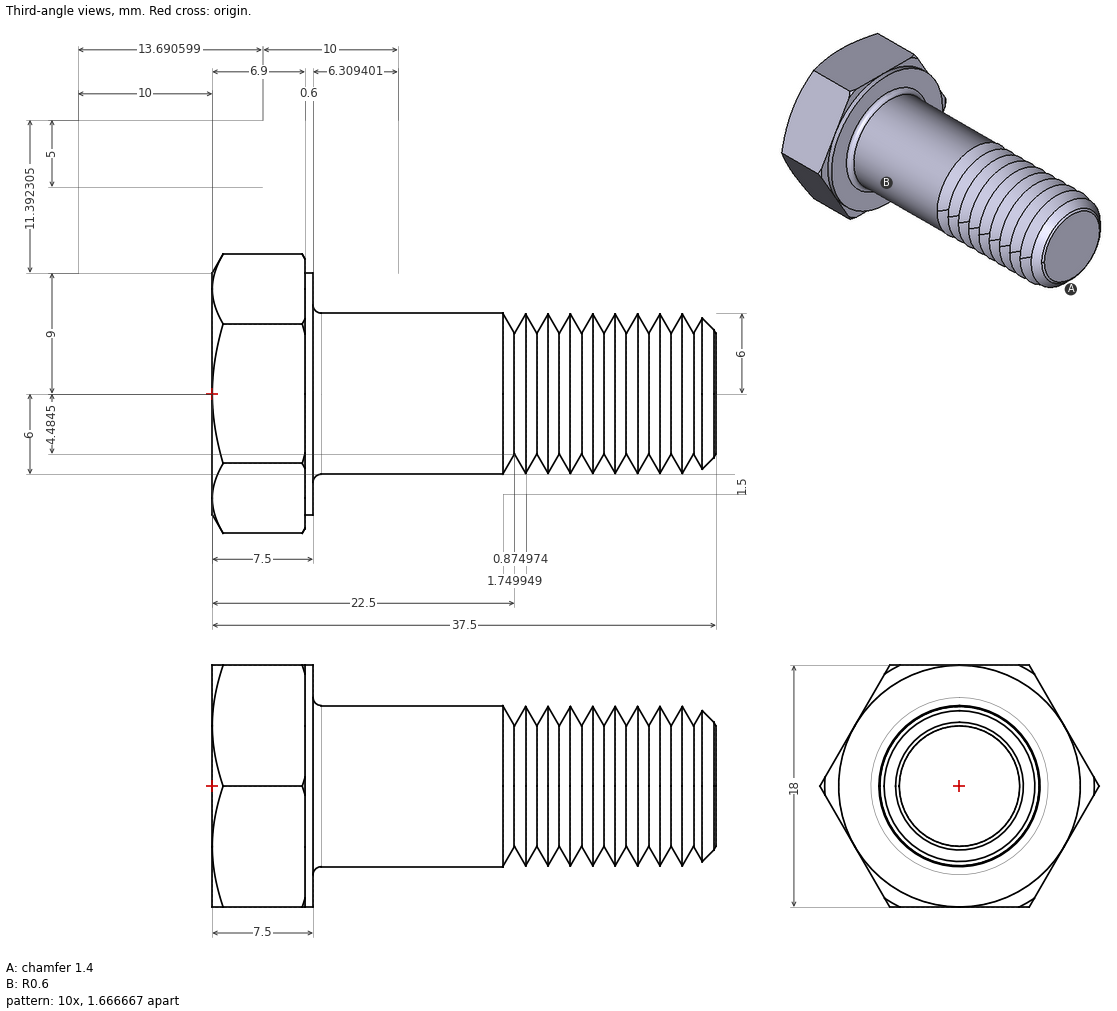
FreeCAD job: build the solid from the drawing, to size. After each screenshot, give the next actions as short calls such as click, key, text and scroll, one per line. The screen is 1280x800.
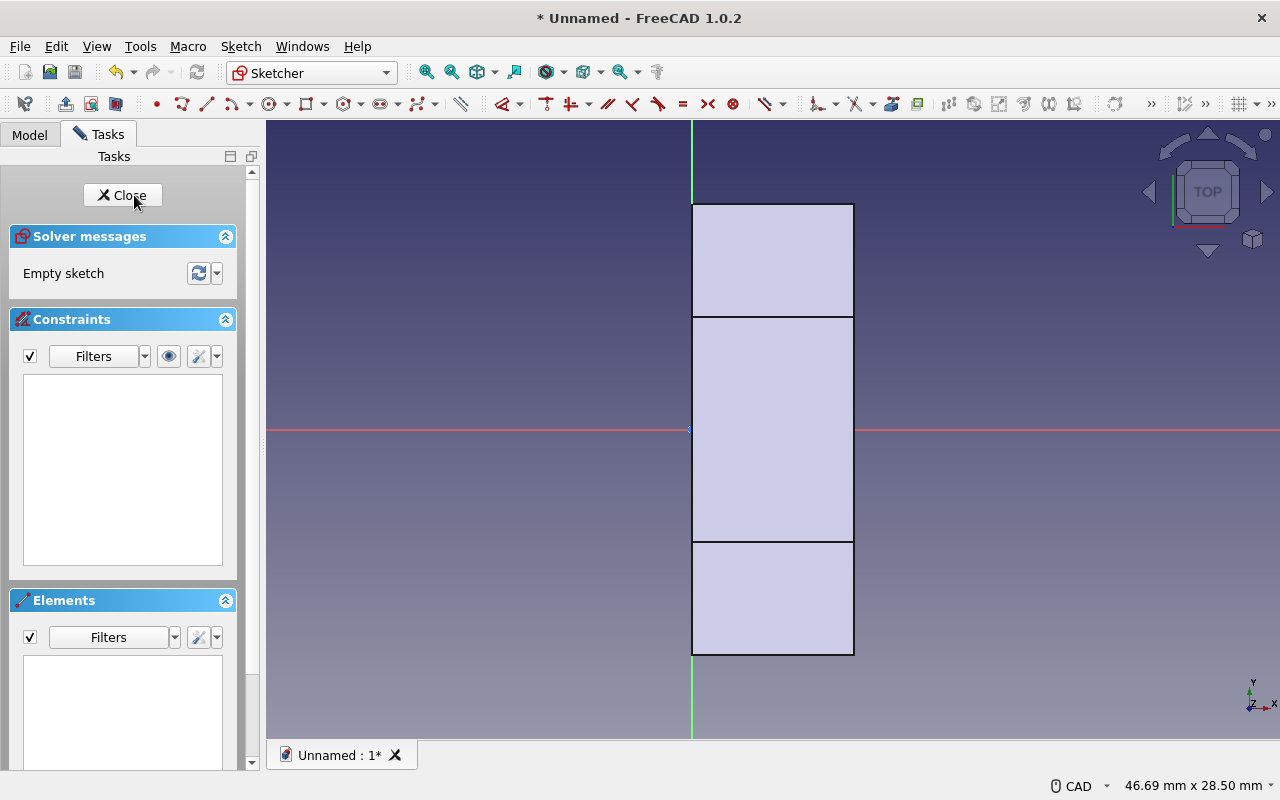
click(116, 104)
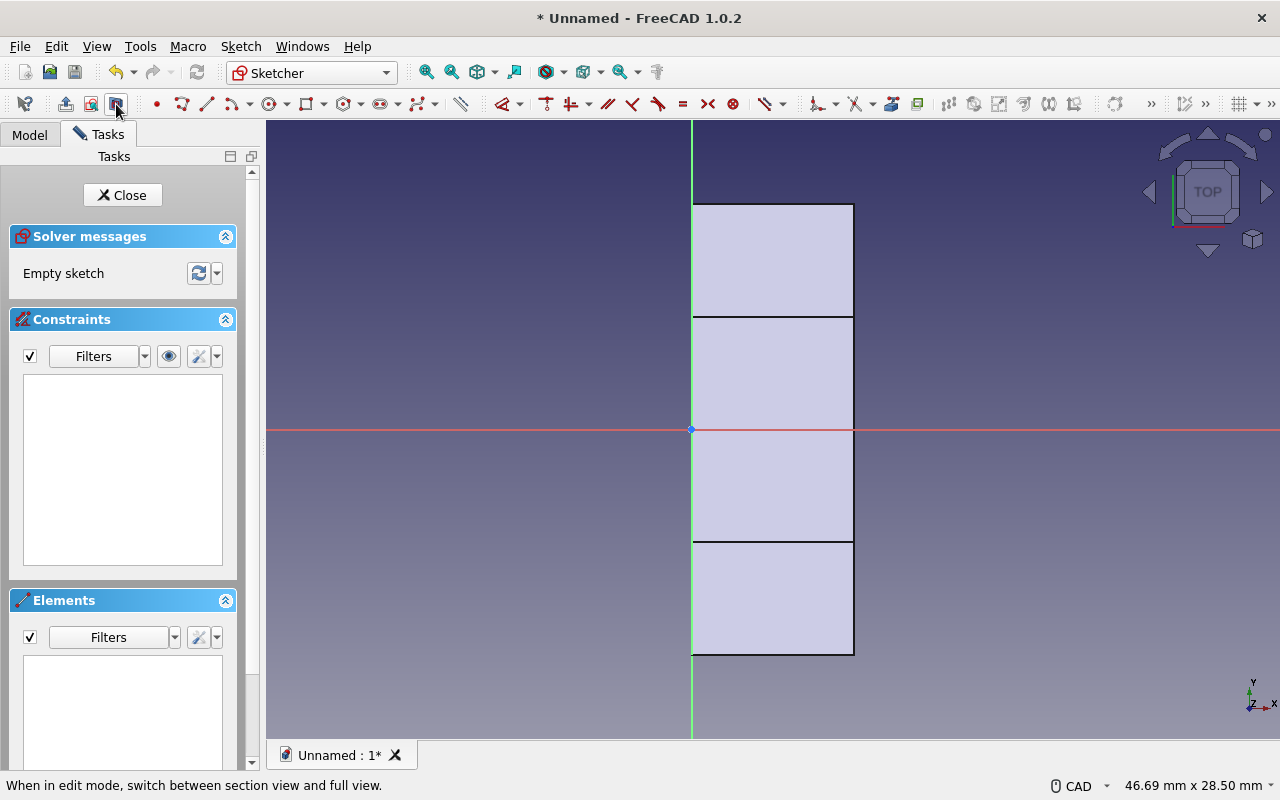
scroll(294, 509, down, 3)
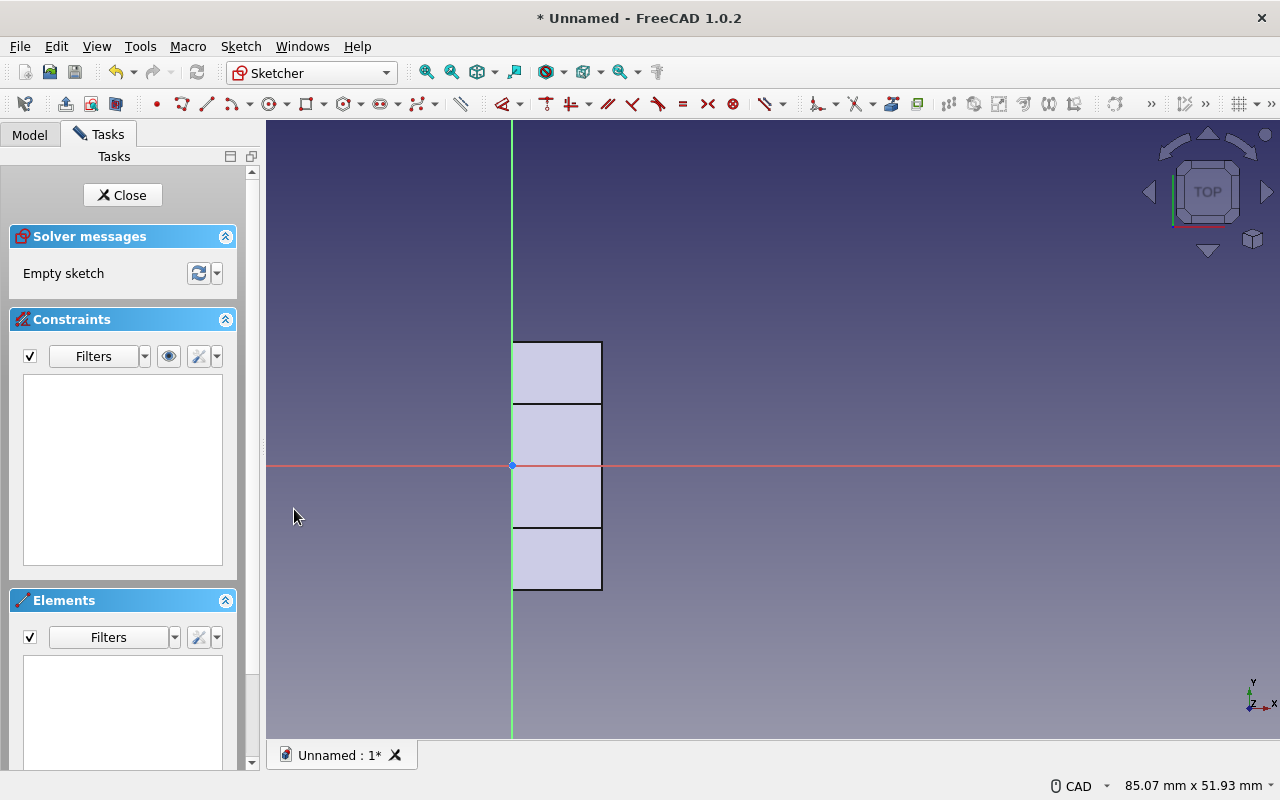
click(306, 104)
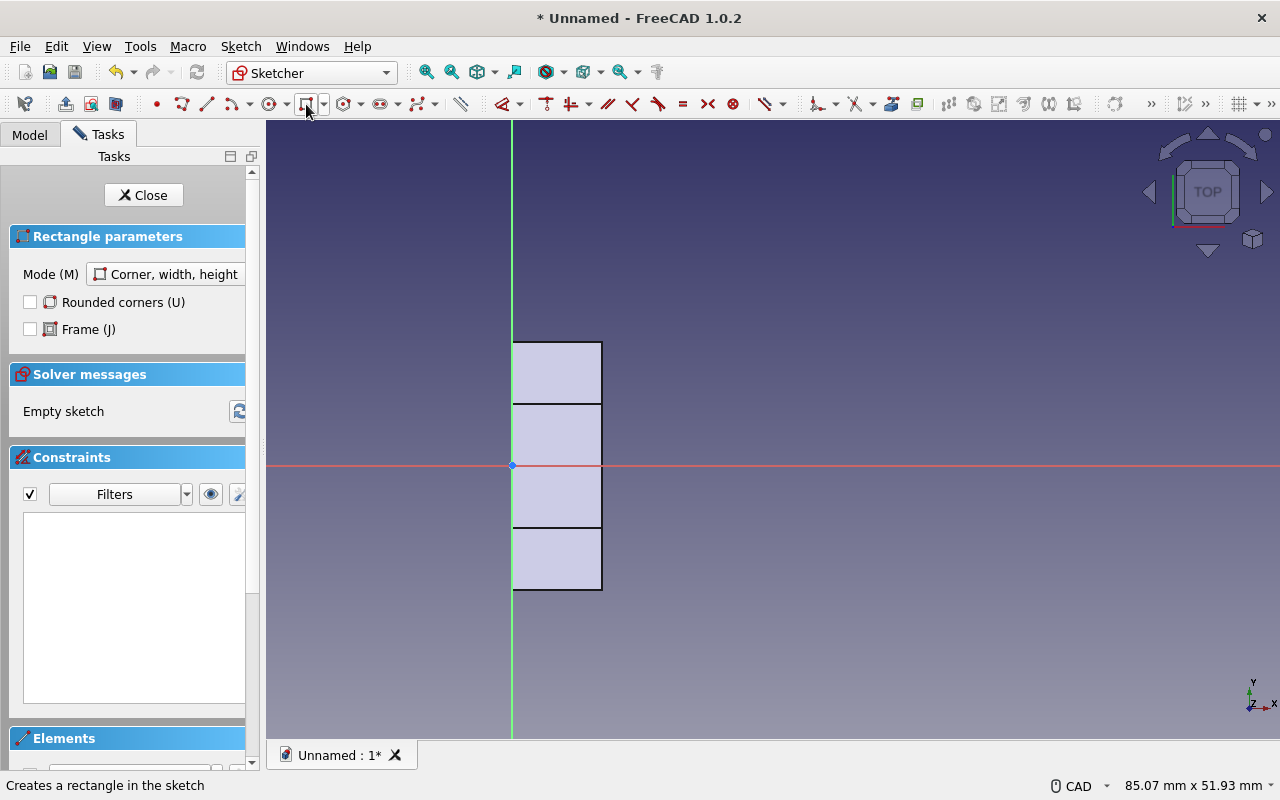
click(512, 466)
click(959, 394)
key(Escape)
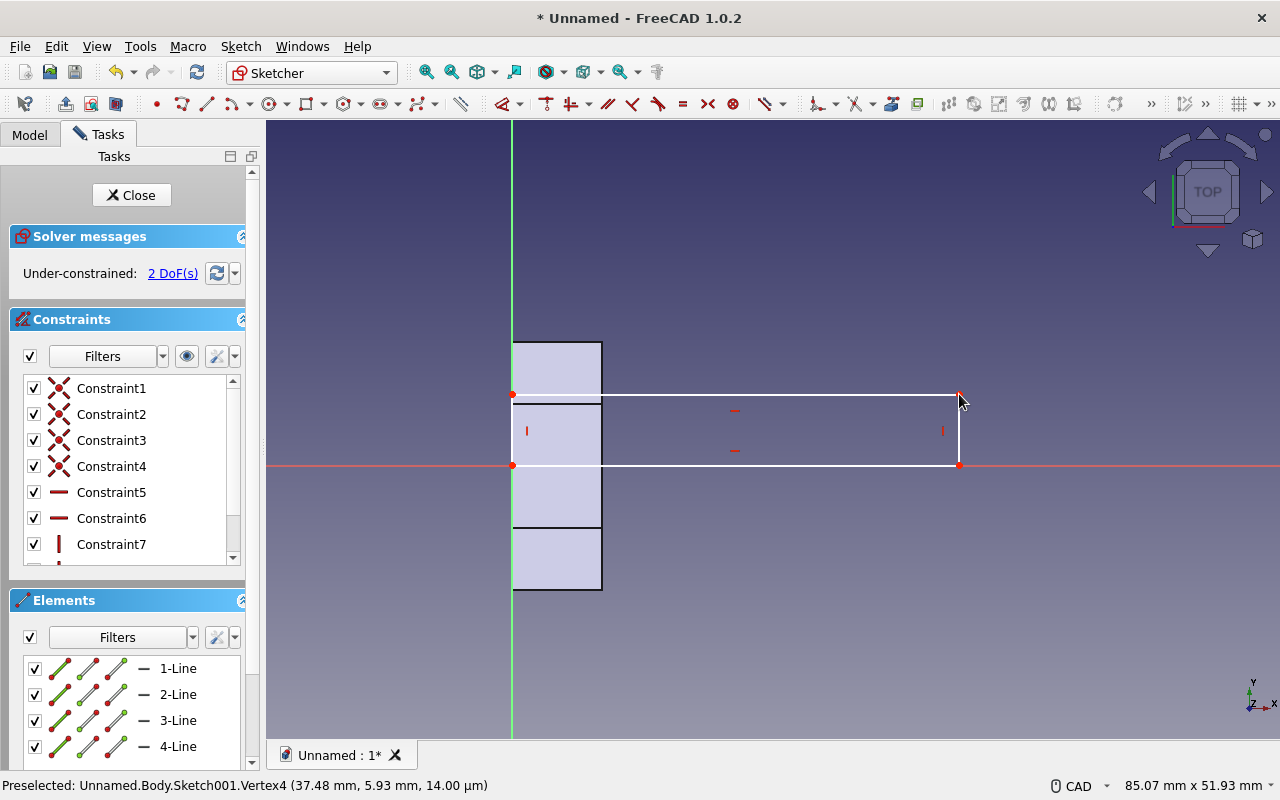
click(959, 444)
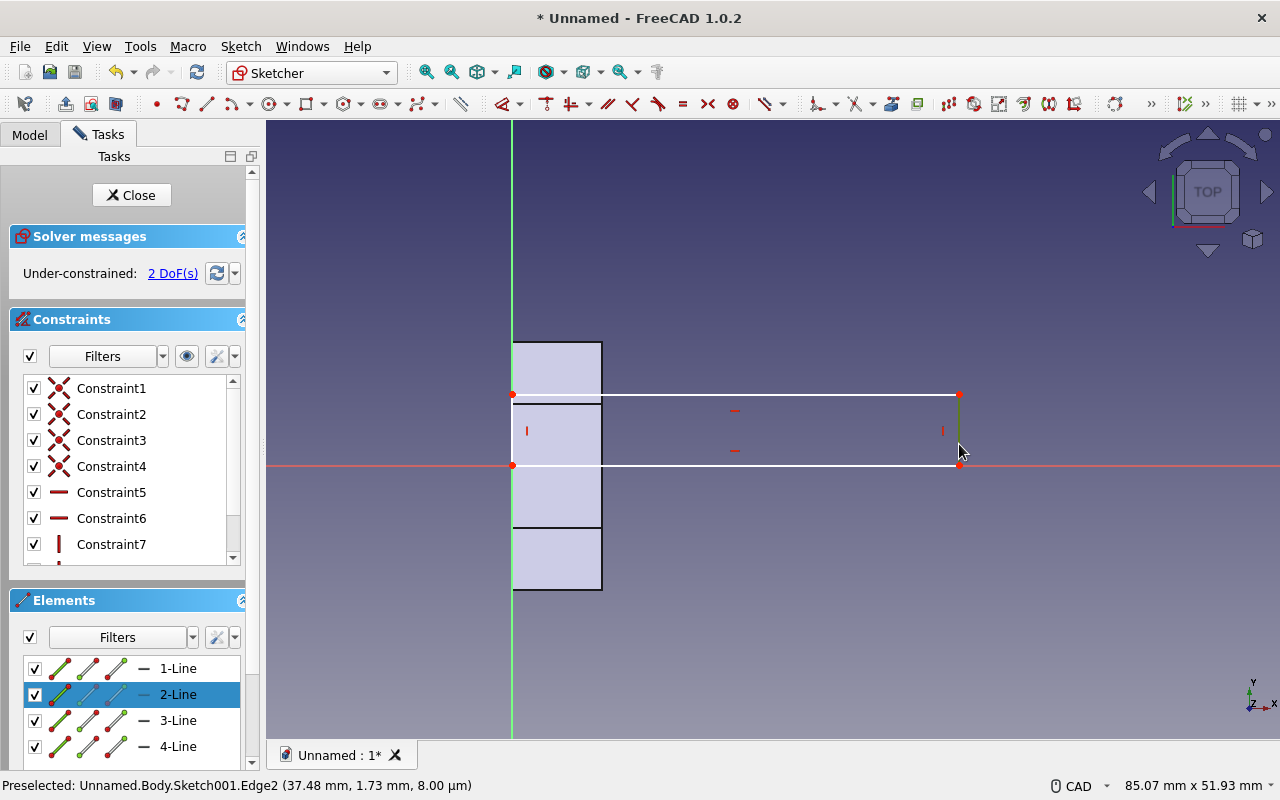
click(520, 104)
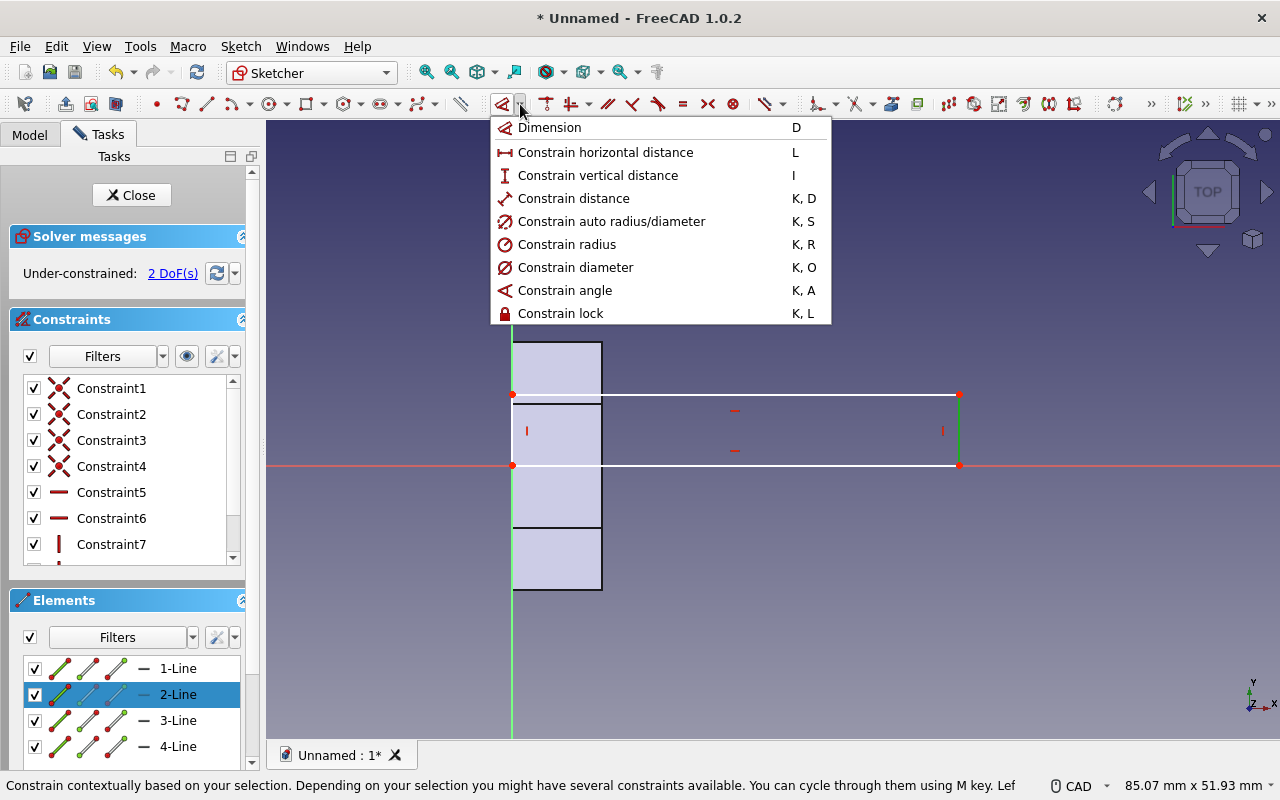
click(661, 176)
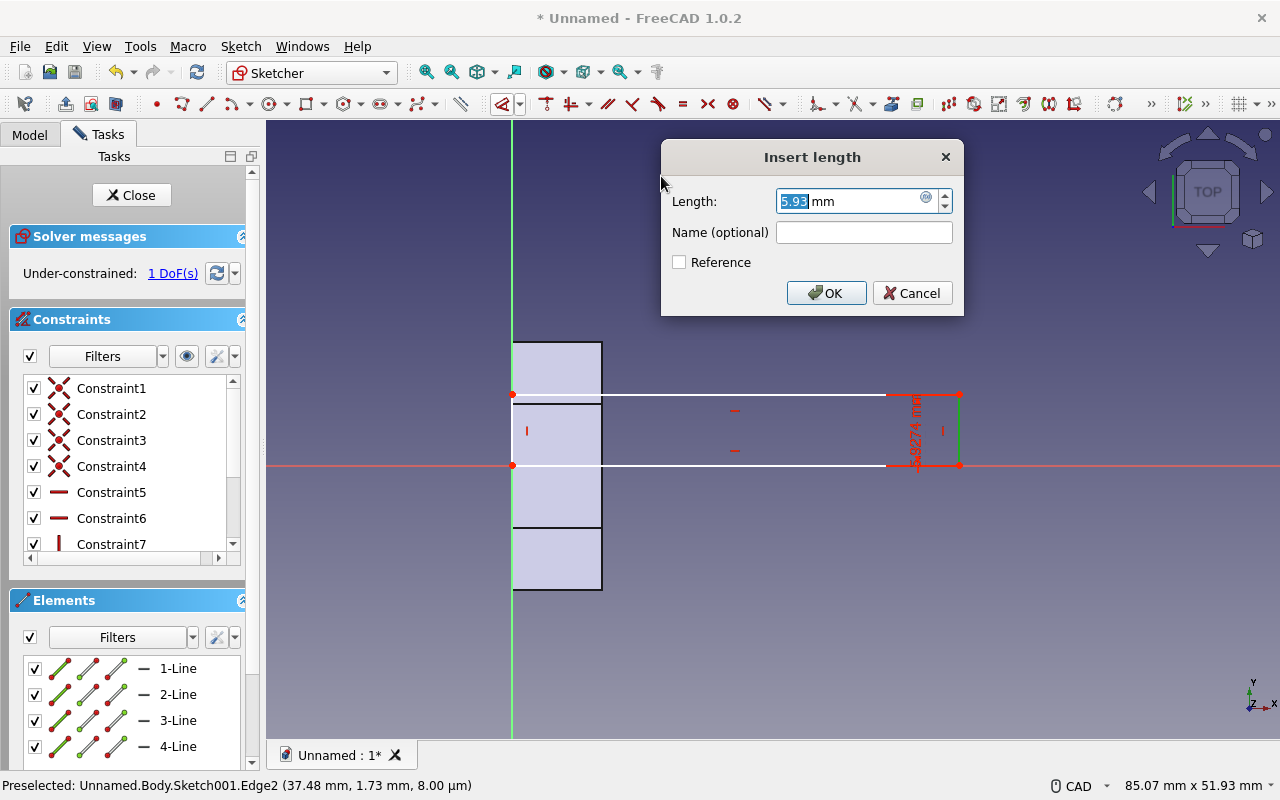
text(6)
key(Return)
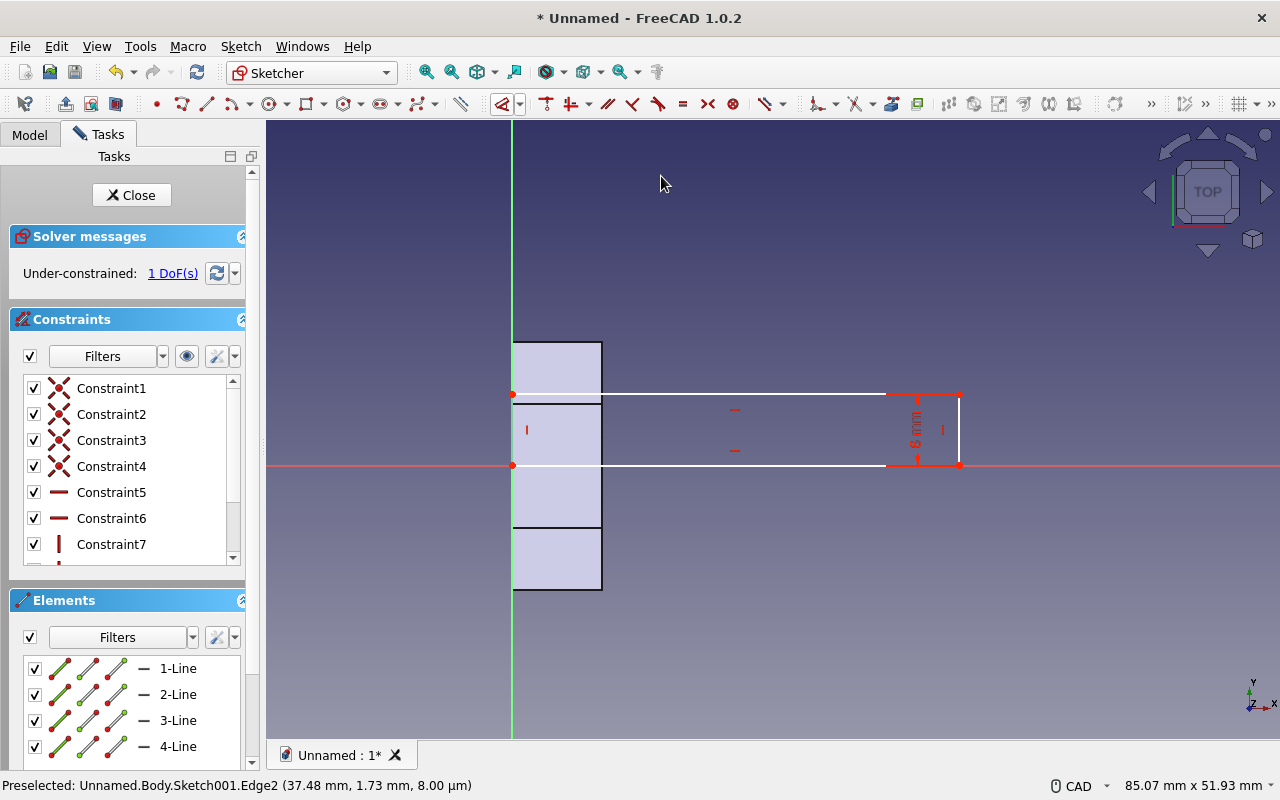
click(646, 466)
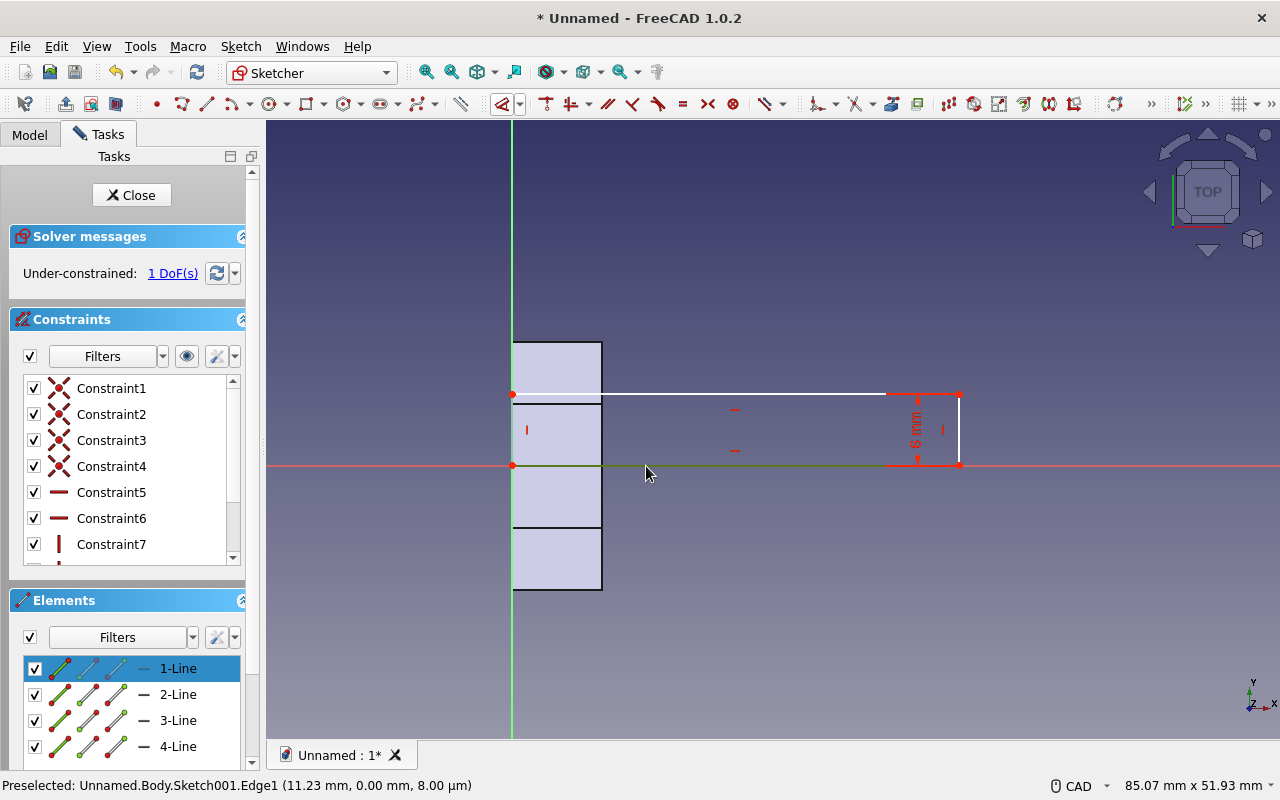
click(520, 104)